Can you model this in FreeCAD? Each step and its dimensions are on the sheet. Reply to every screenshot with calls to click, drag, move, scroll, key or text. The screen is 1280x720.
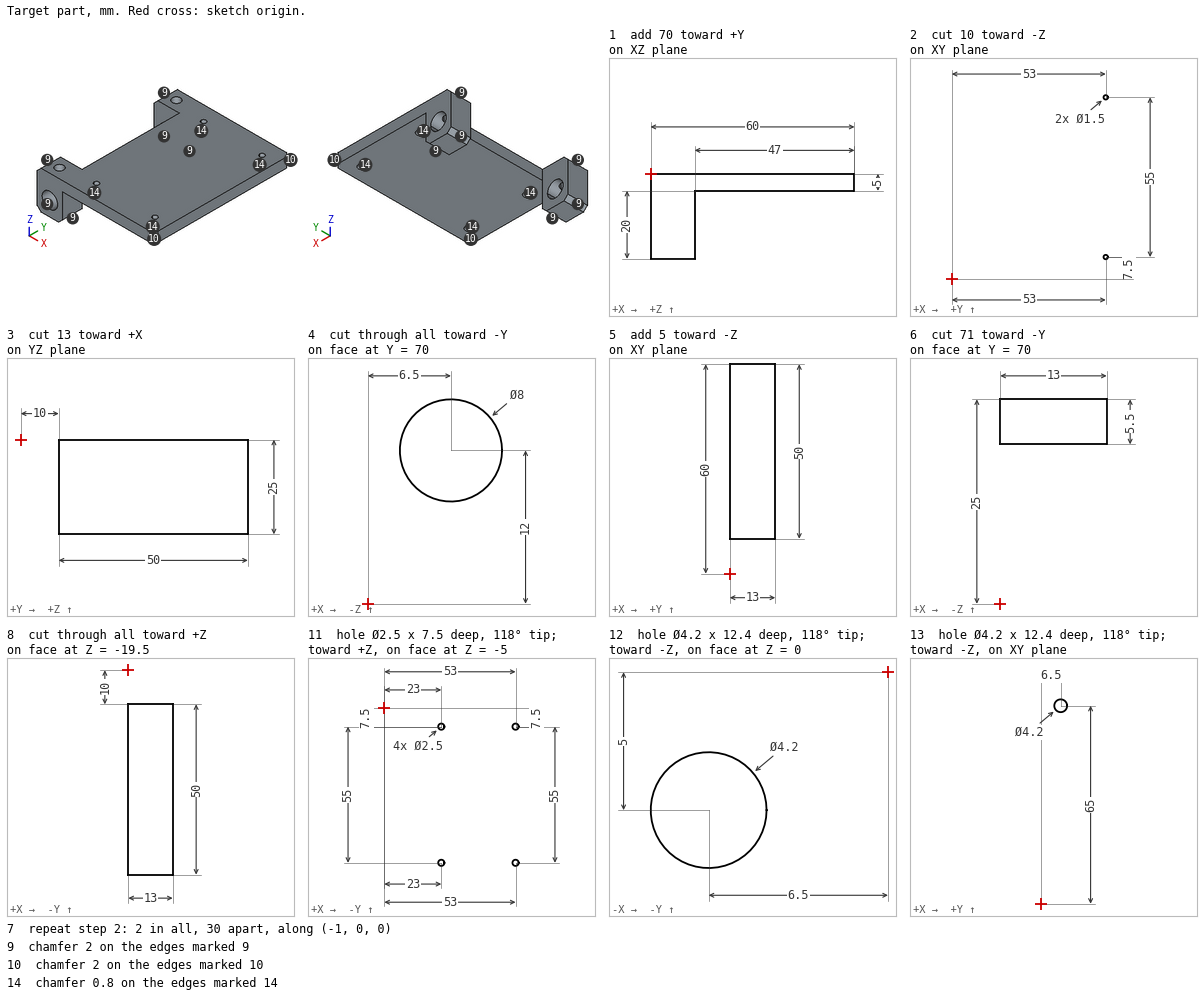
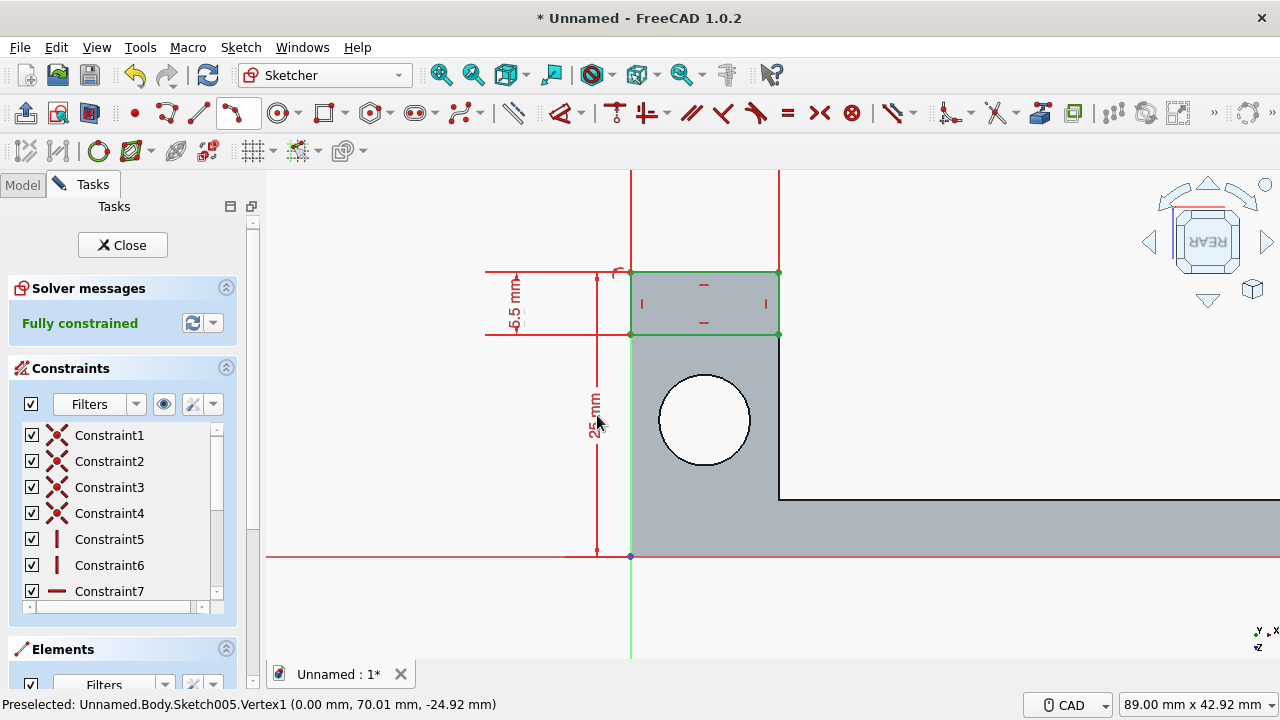
click(123, 245)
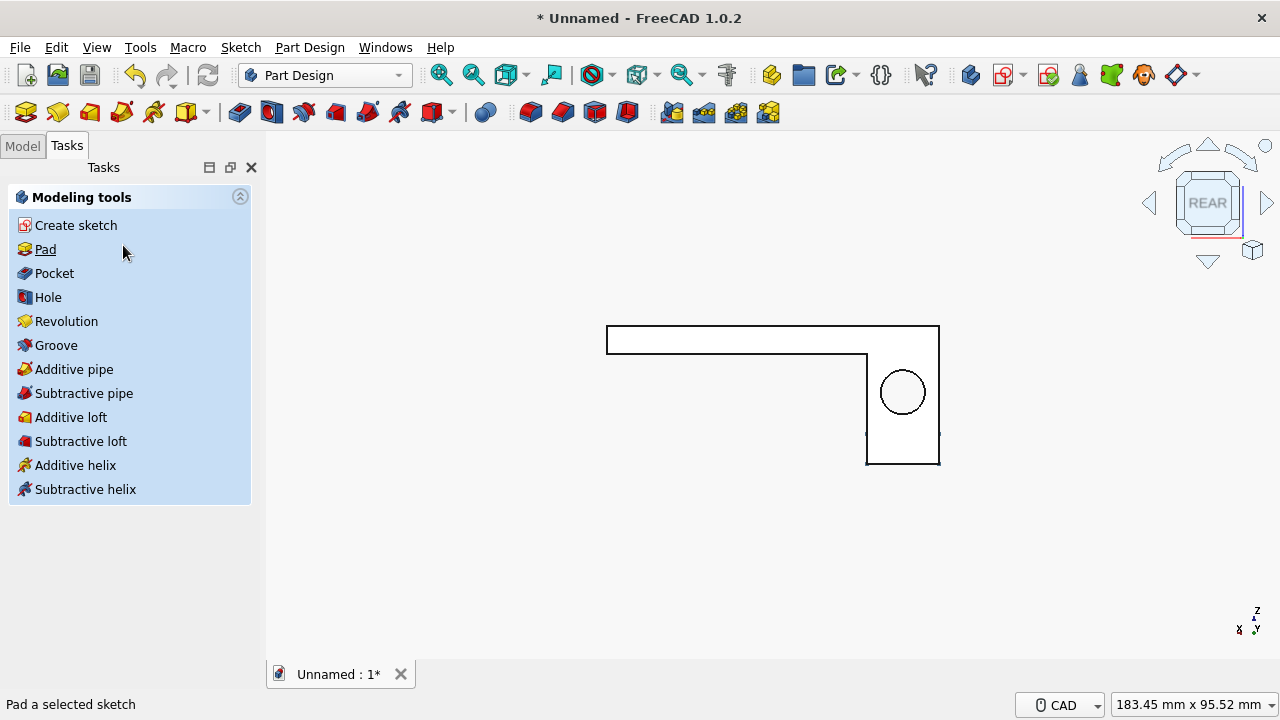
click(240, 112)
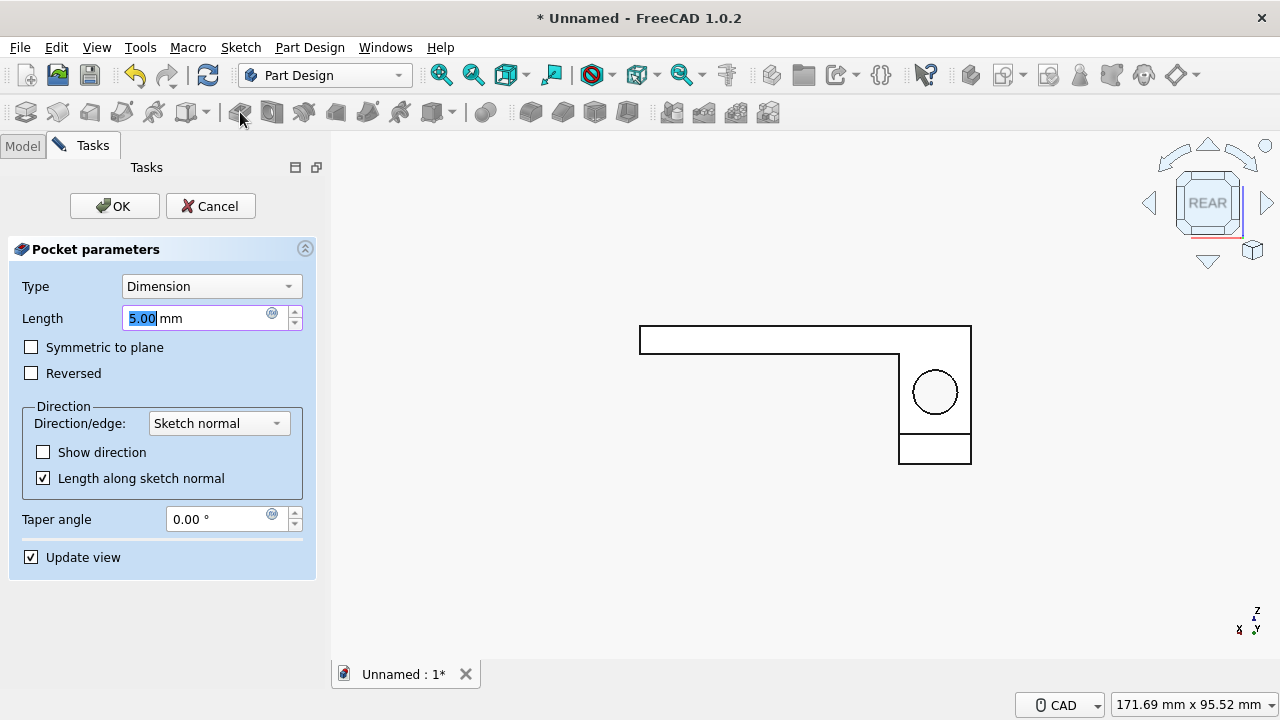
text(71)
key(Tab)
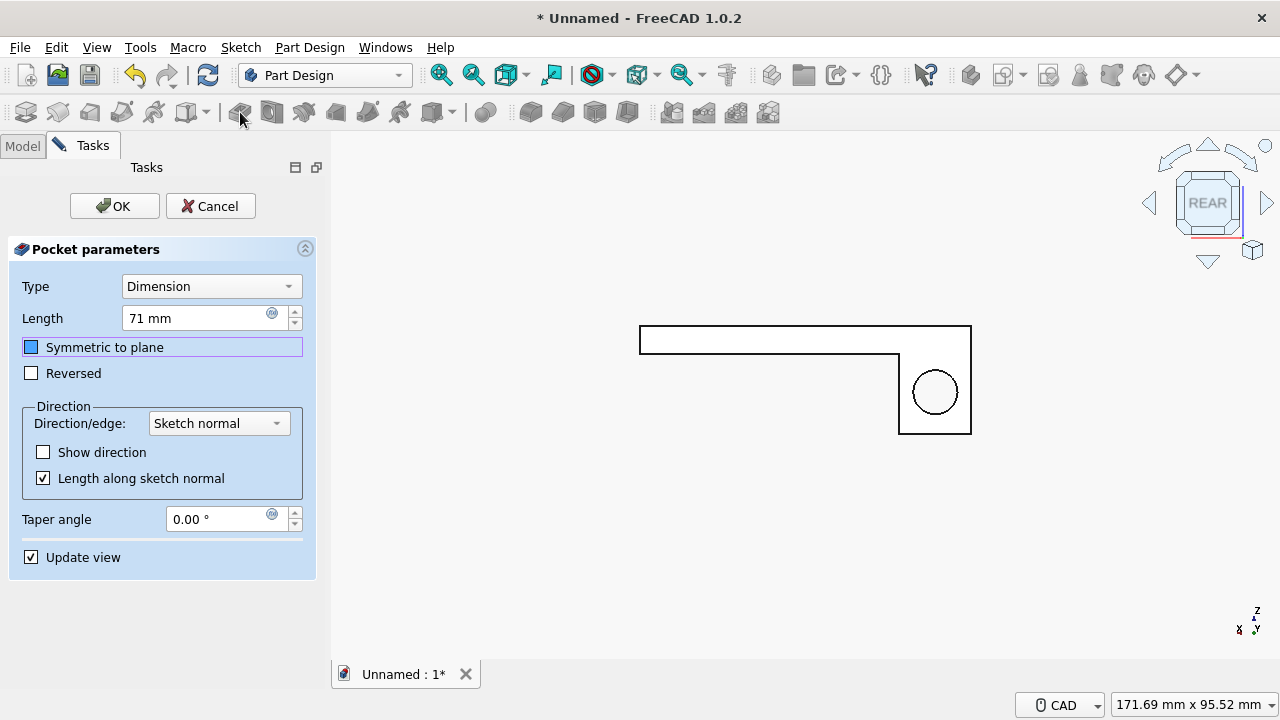
click(115, 206)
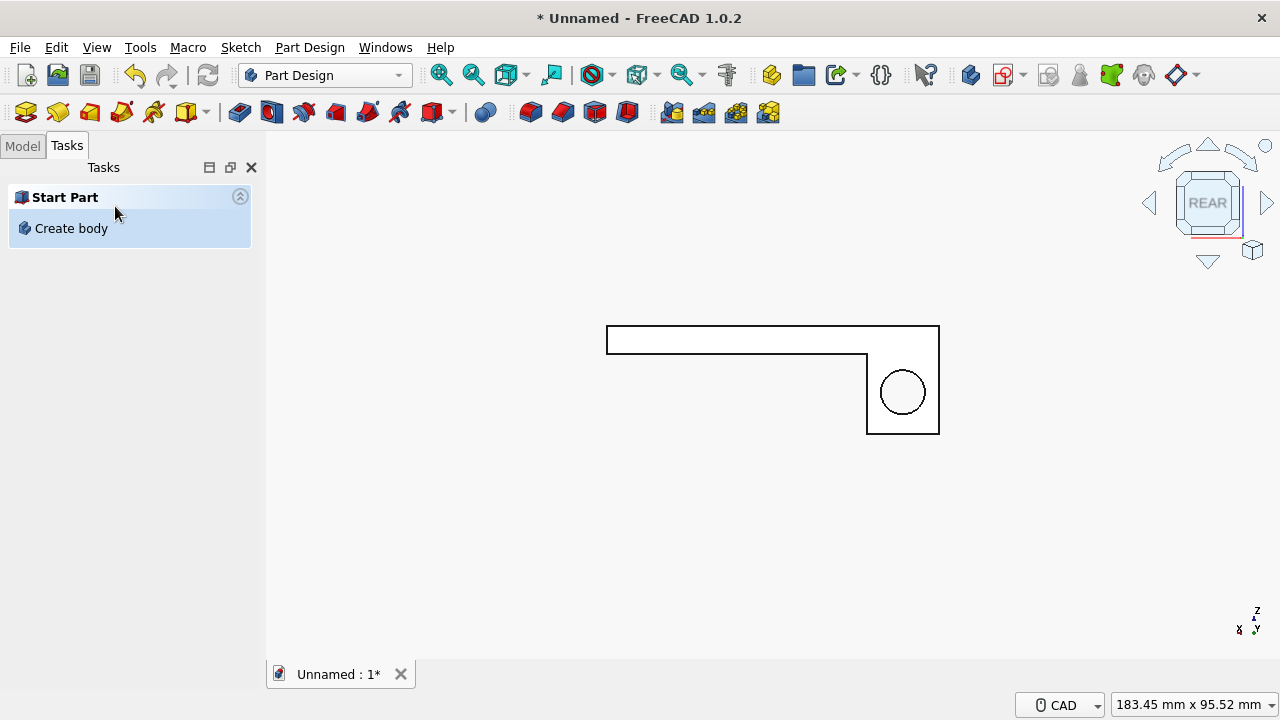
click(442, 76)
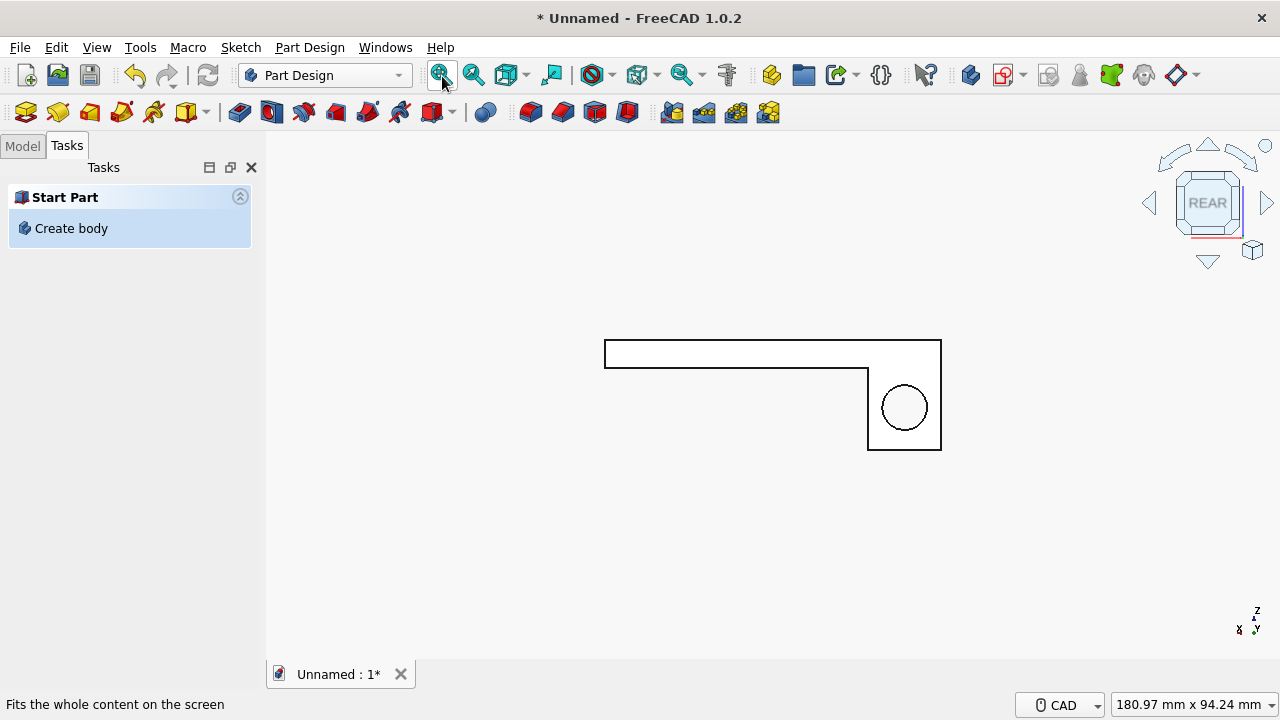
click(23, 145)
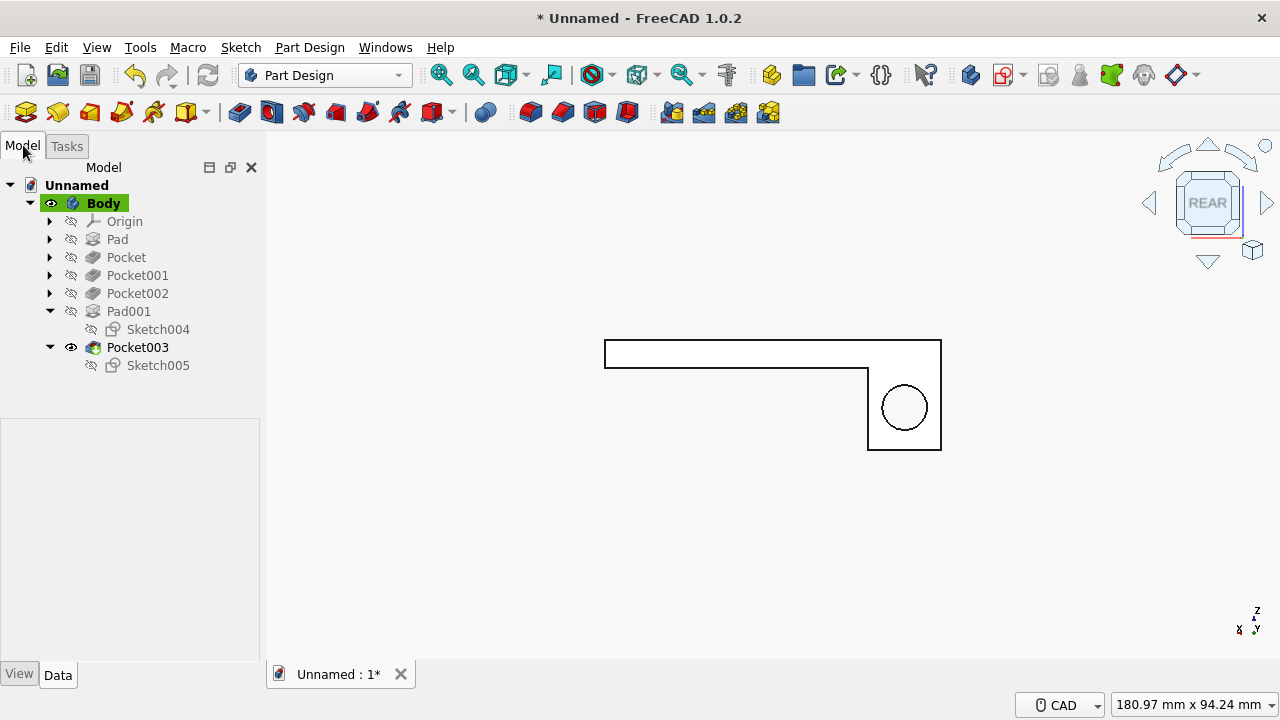
click(116, 257)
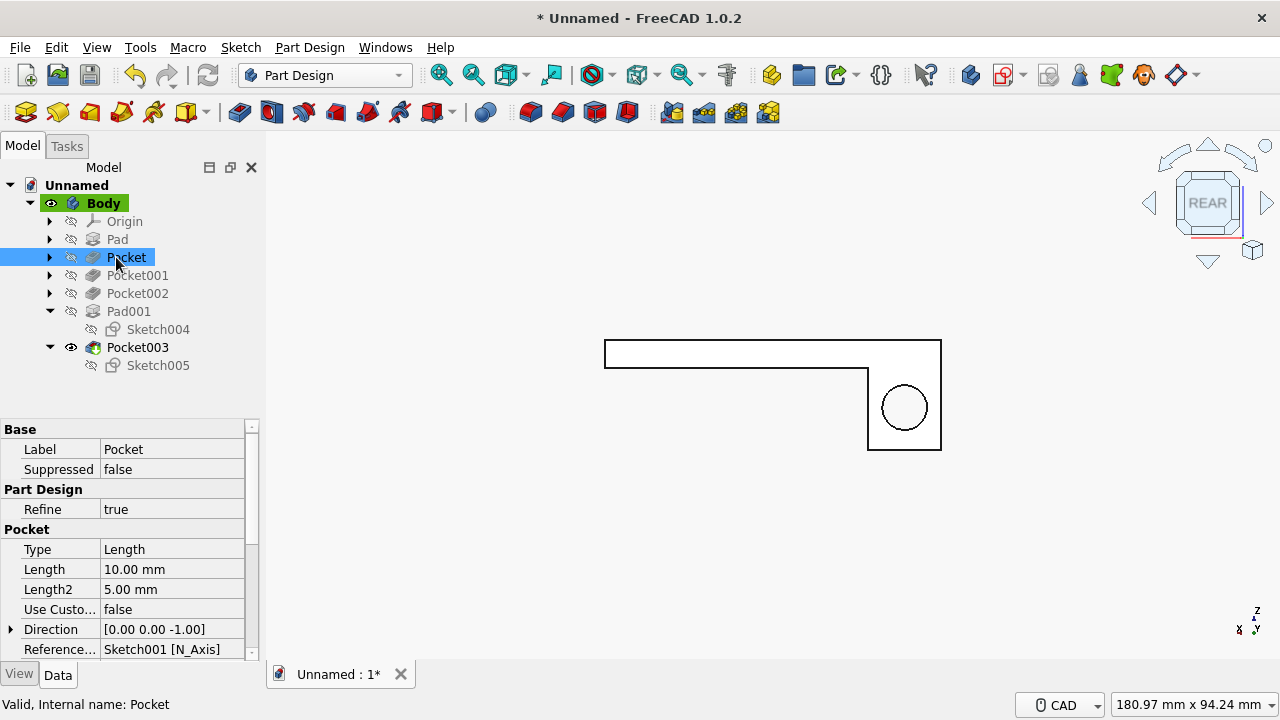
click(704, 112)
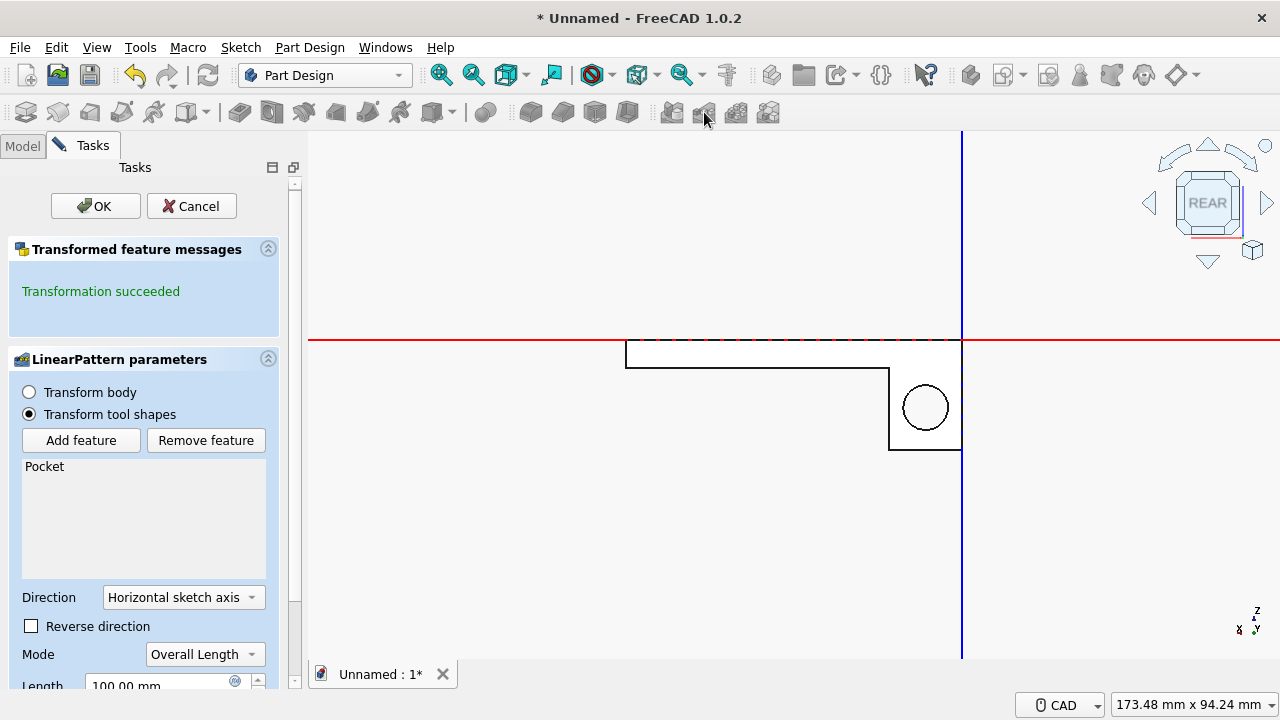
click(184, 598)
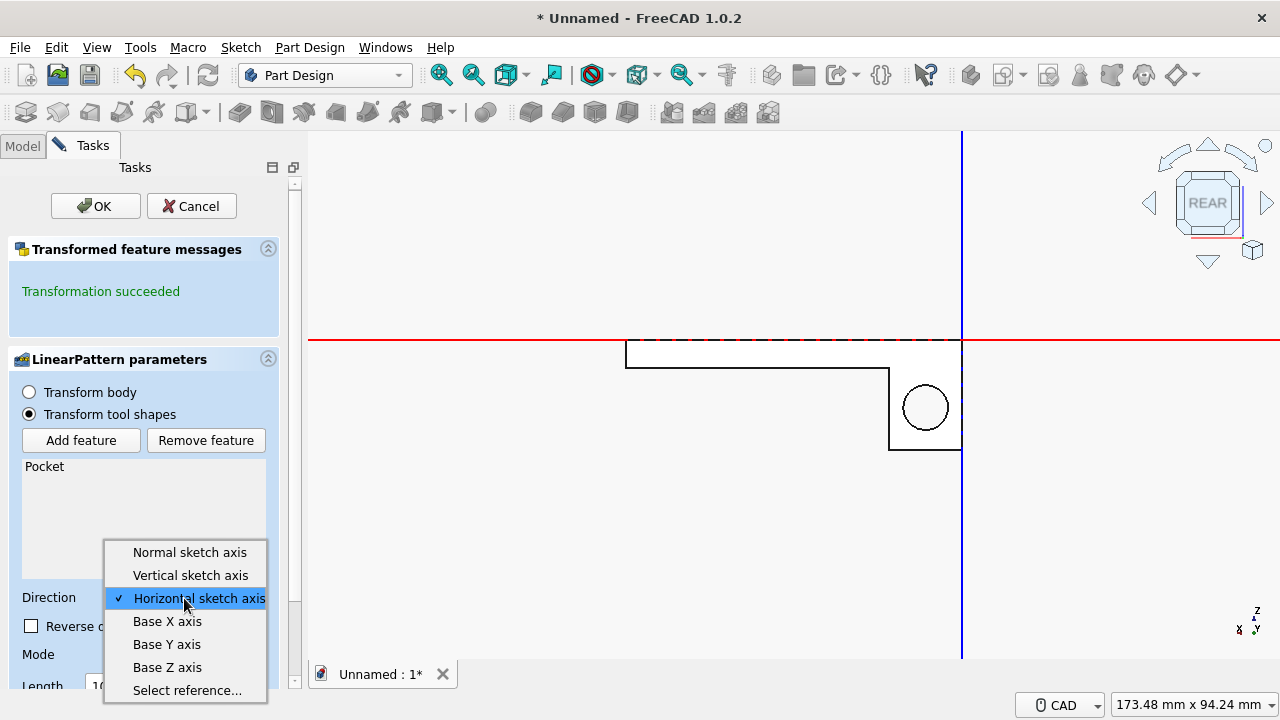
click(184, 622)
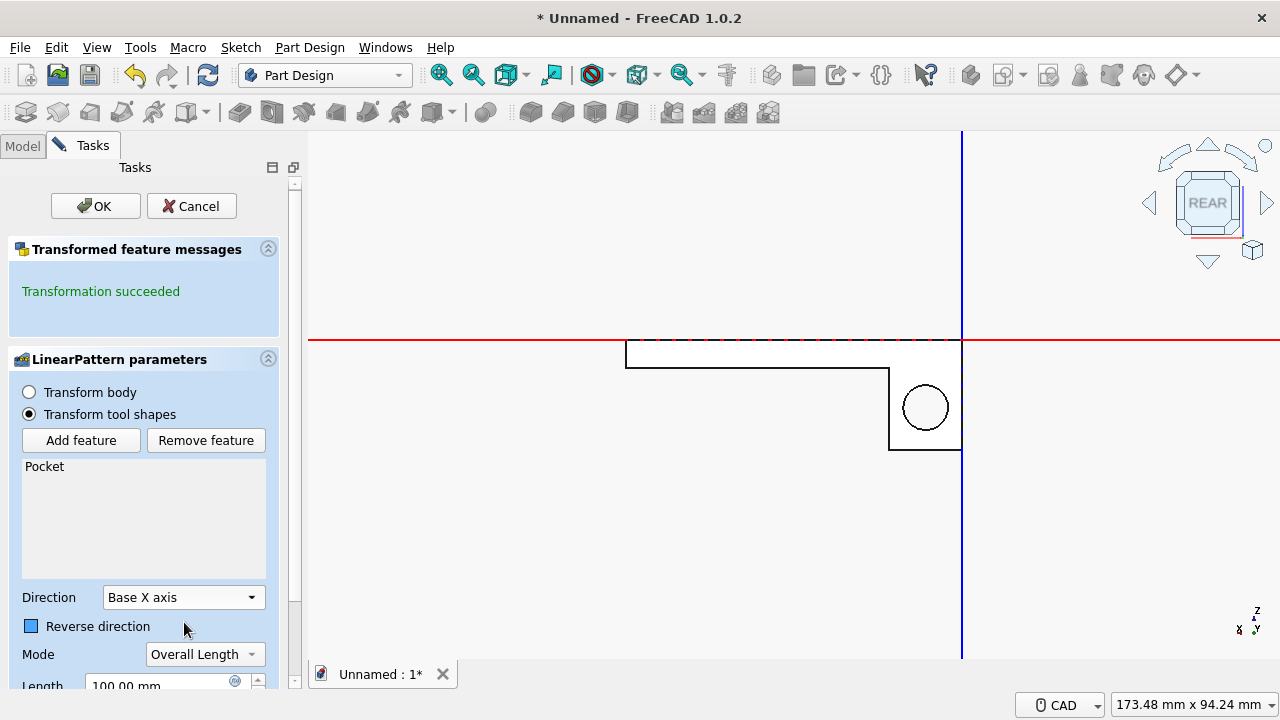
click(206, 654)